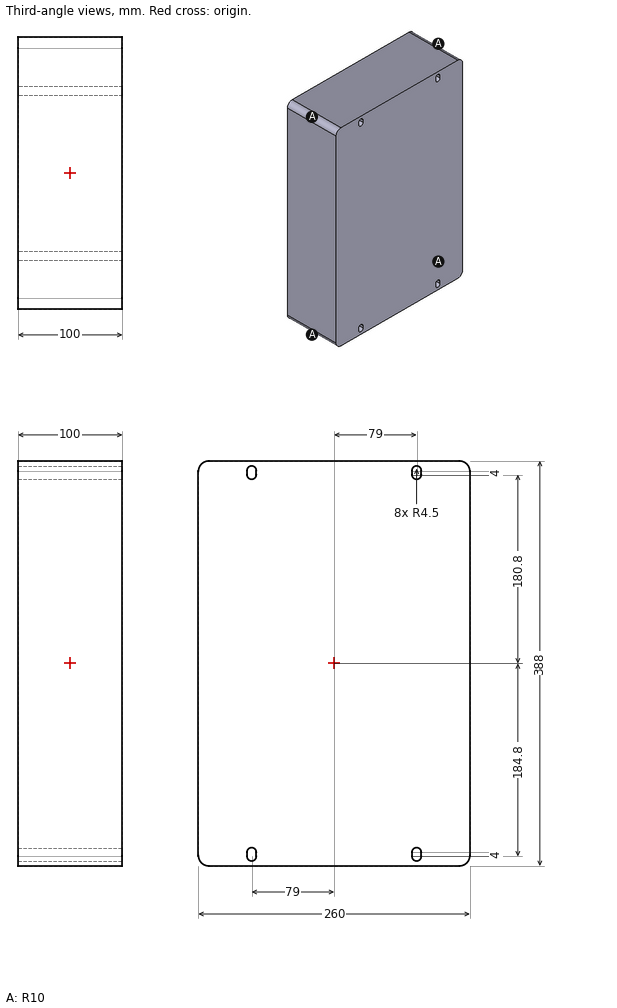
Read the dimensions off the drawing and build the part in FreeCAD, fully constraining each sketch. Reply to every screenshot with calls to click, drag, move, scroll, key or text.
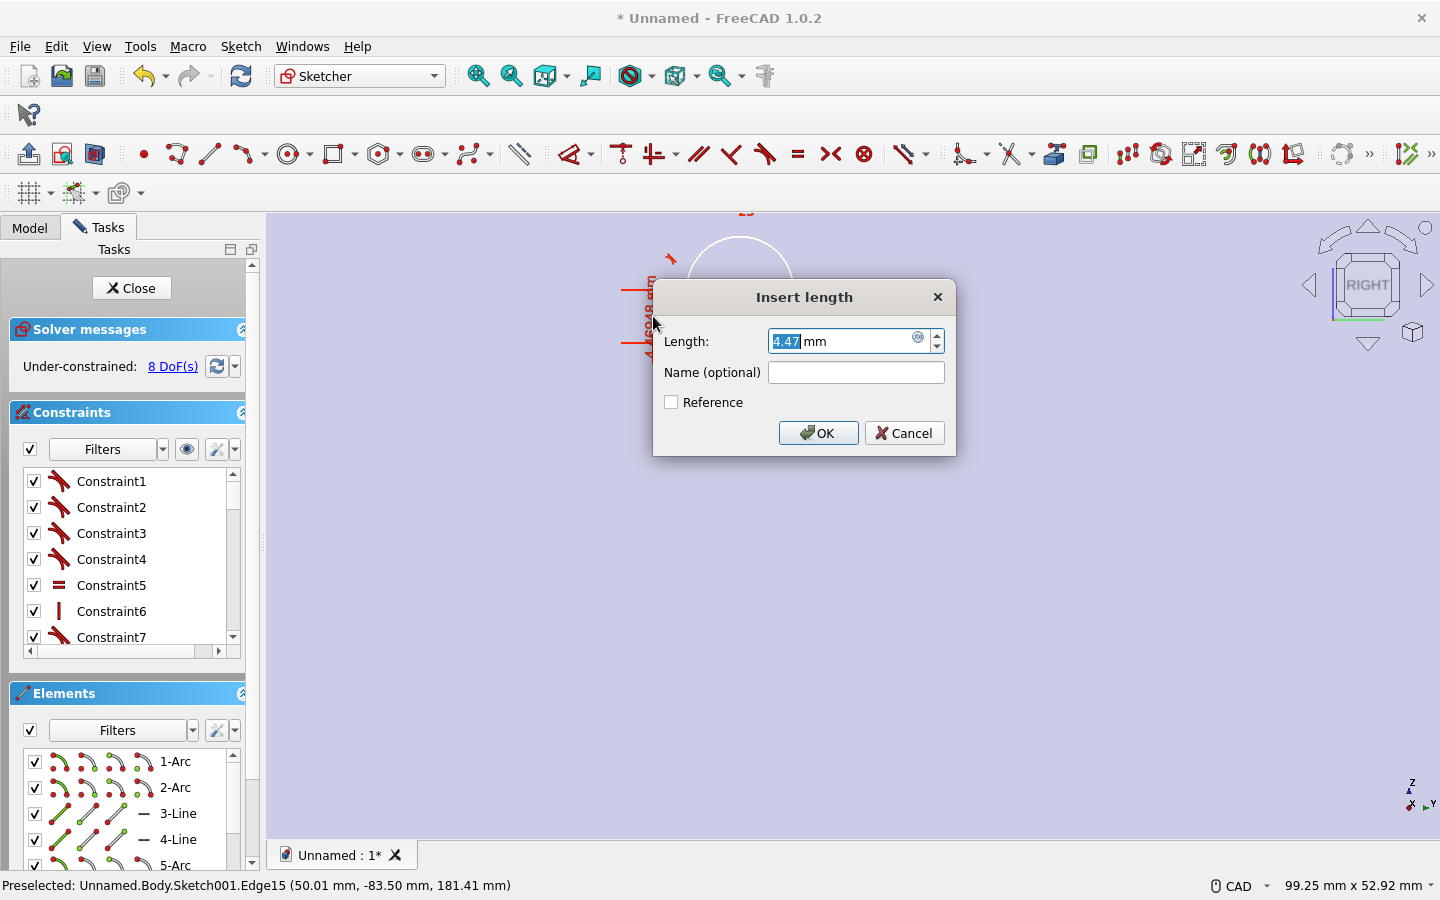
text(4)
key(Return)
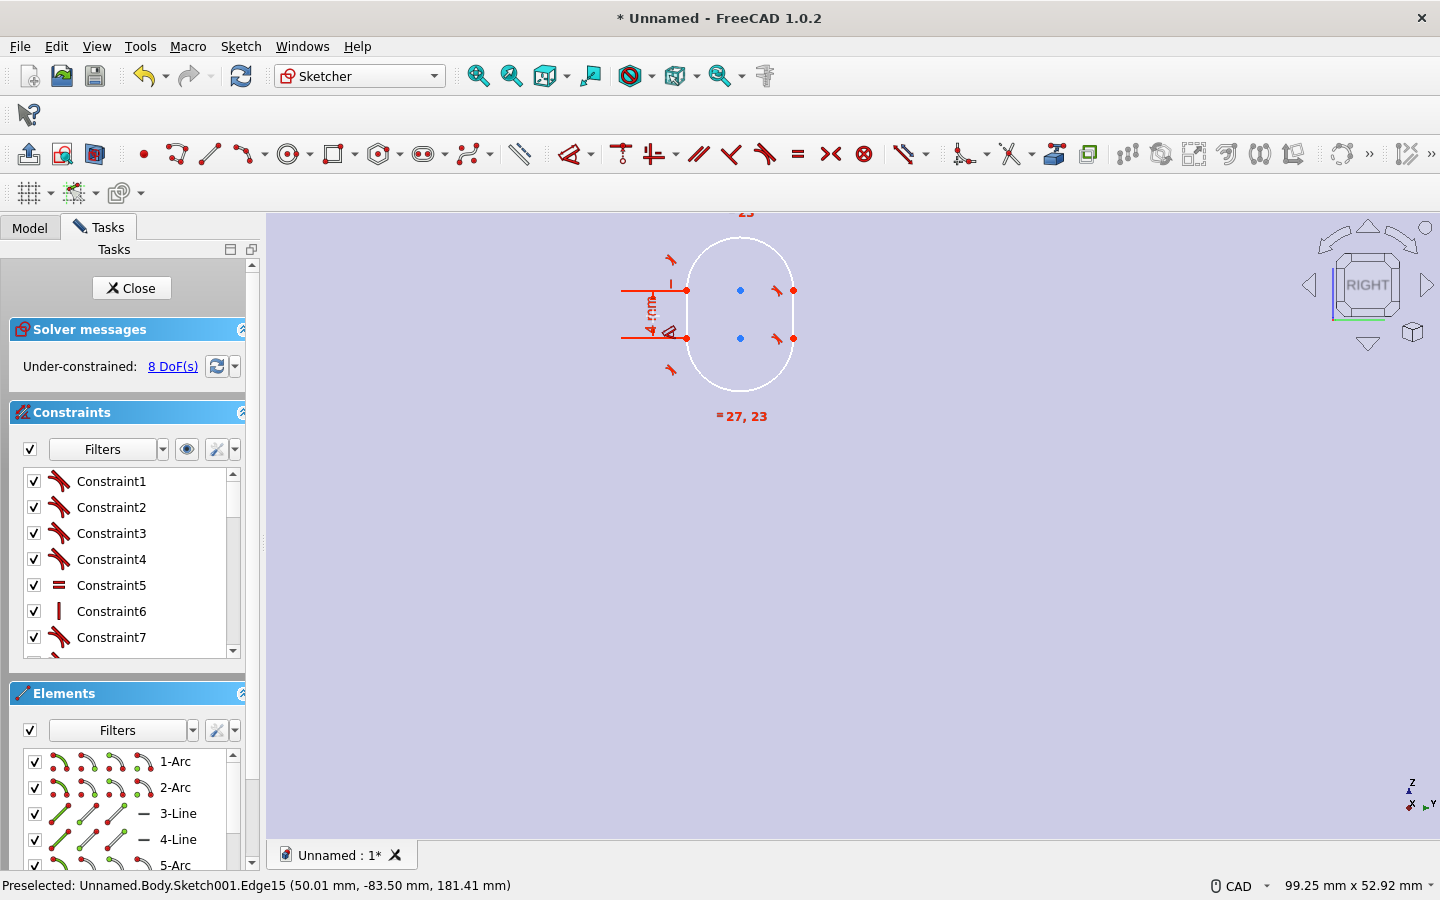
scroll(696, 332, down, 12)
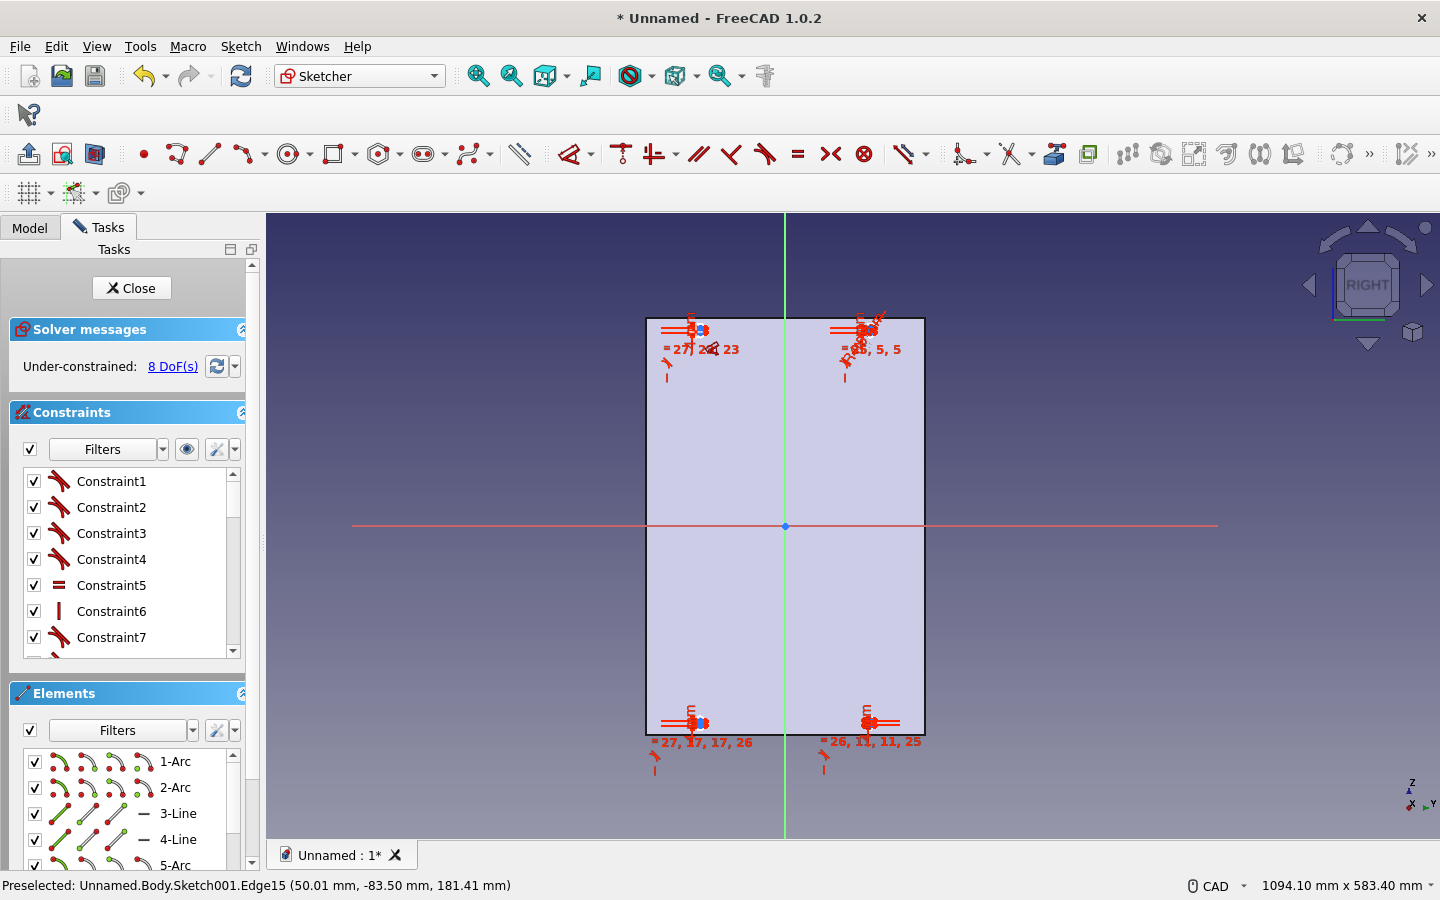
scroll(870, 333, up, 6)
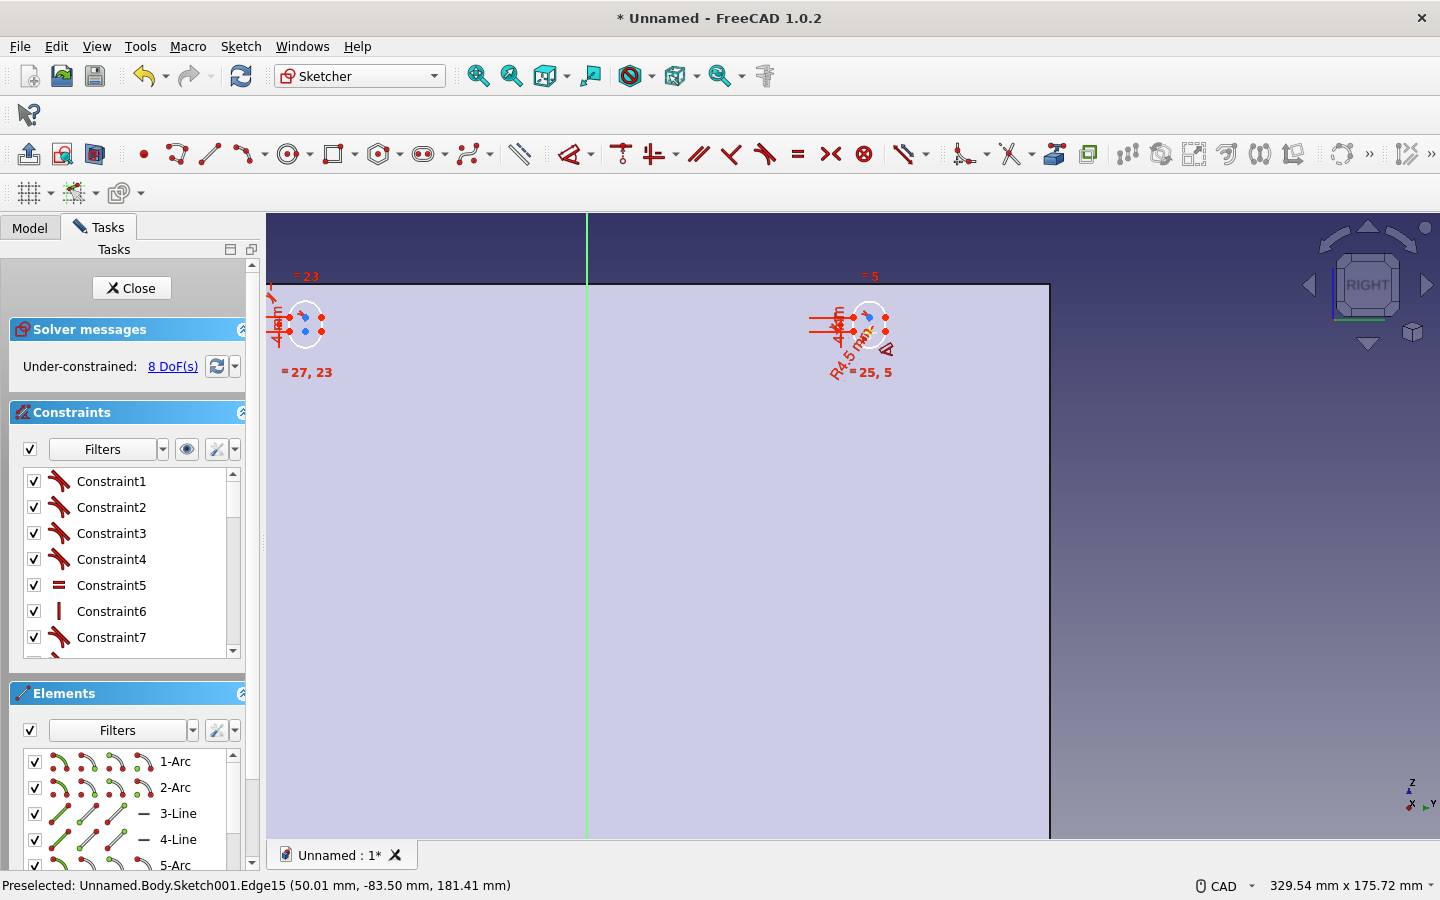
click(869, 332)
click(728, 298)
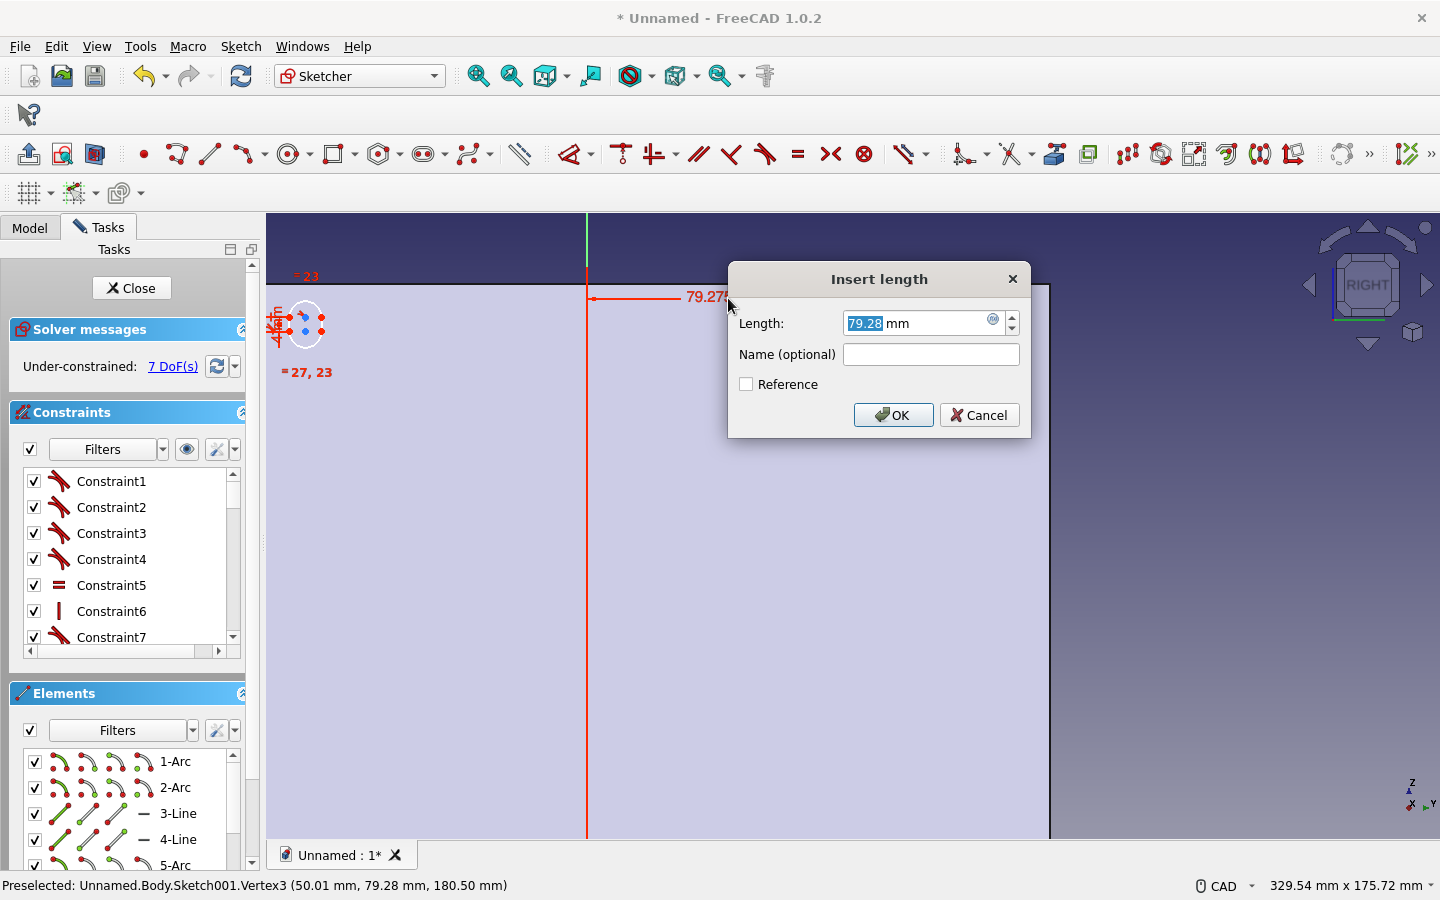
text(79)
key(Return)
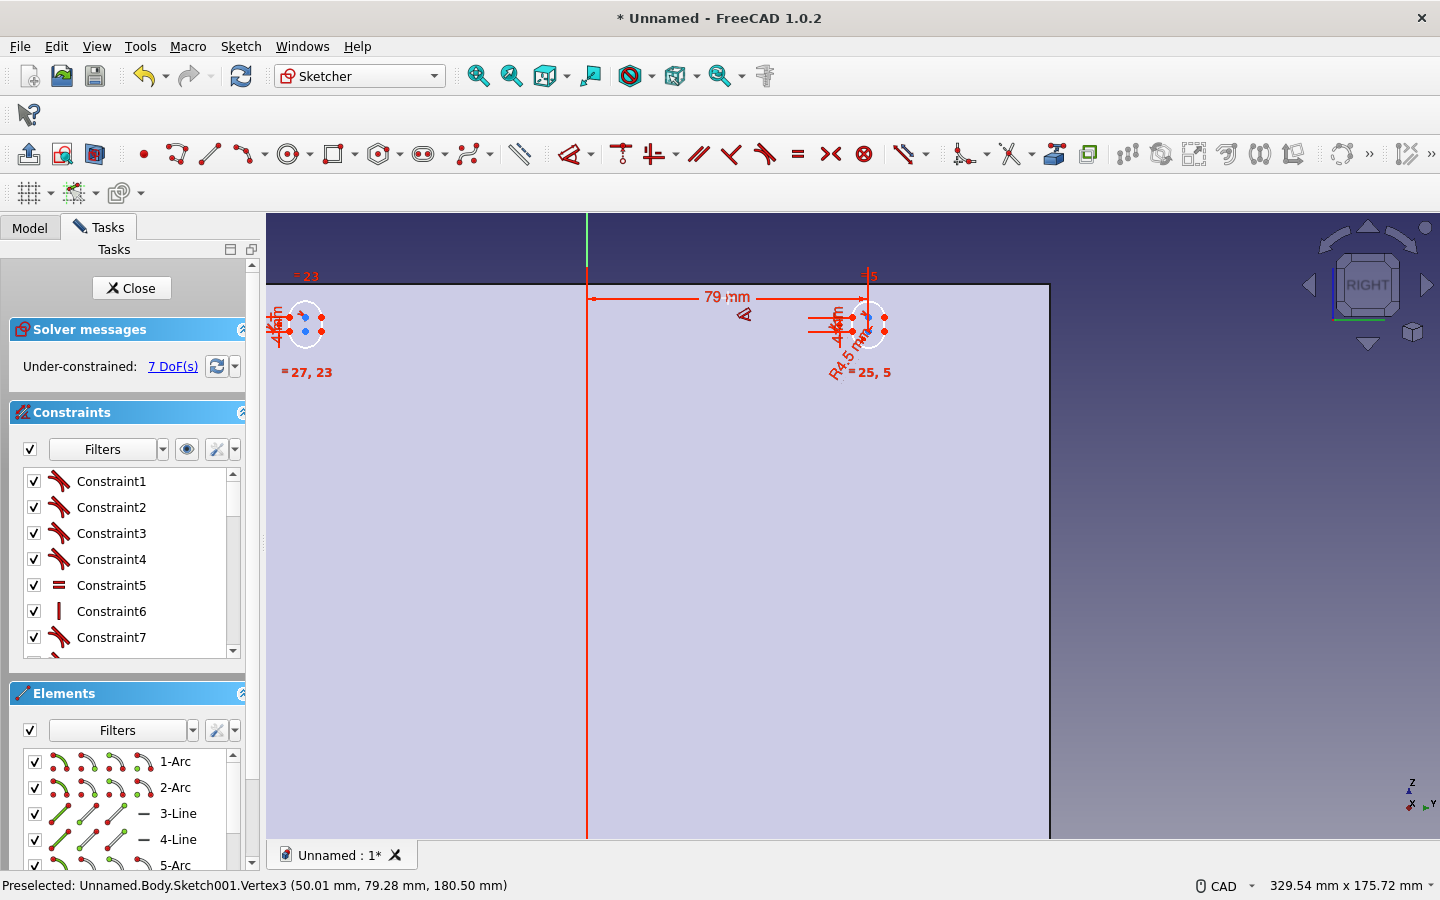
scroll(870, 333, down, 6)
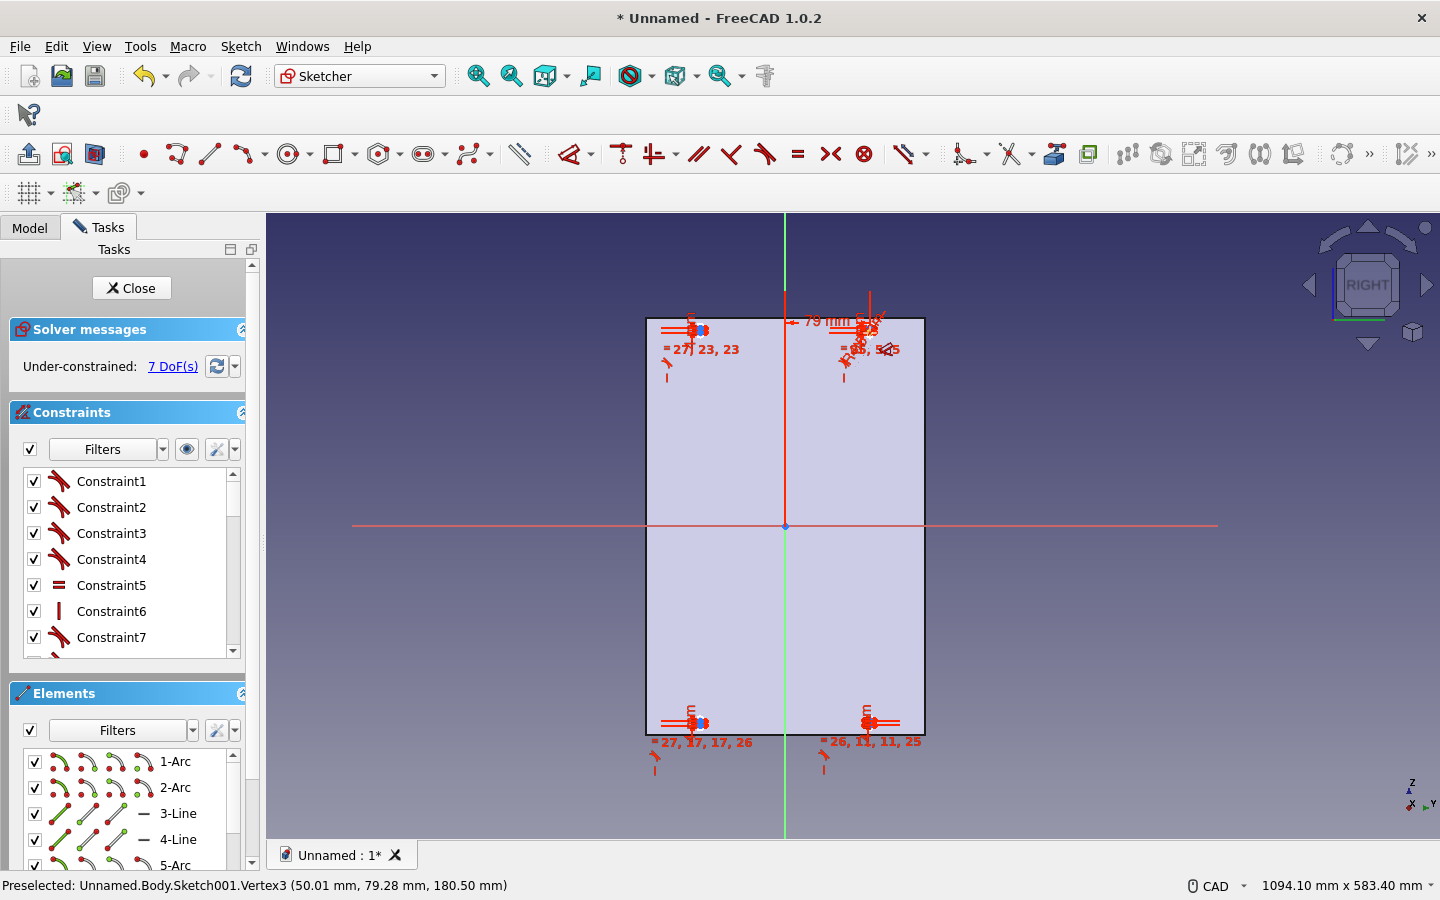
scroll(870, 725, up, 6)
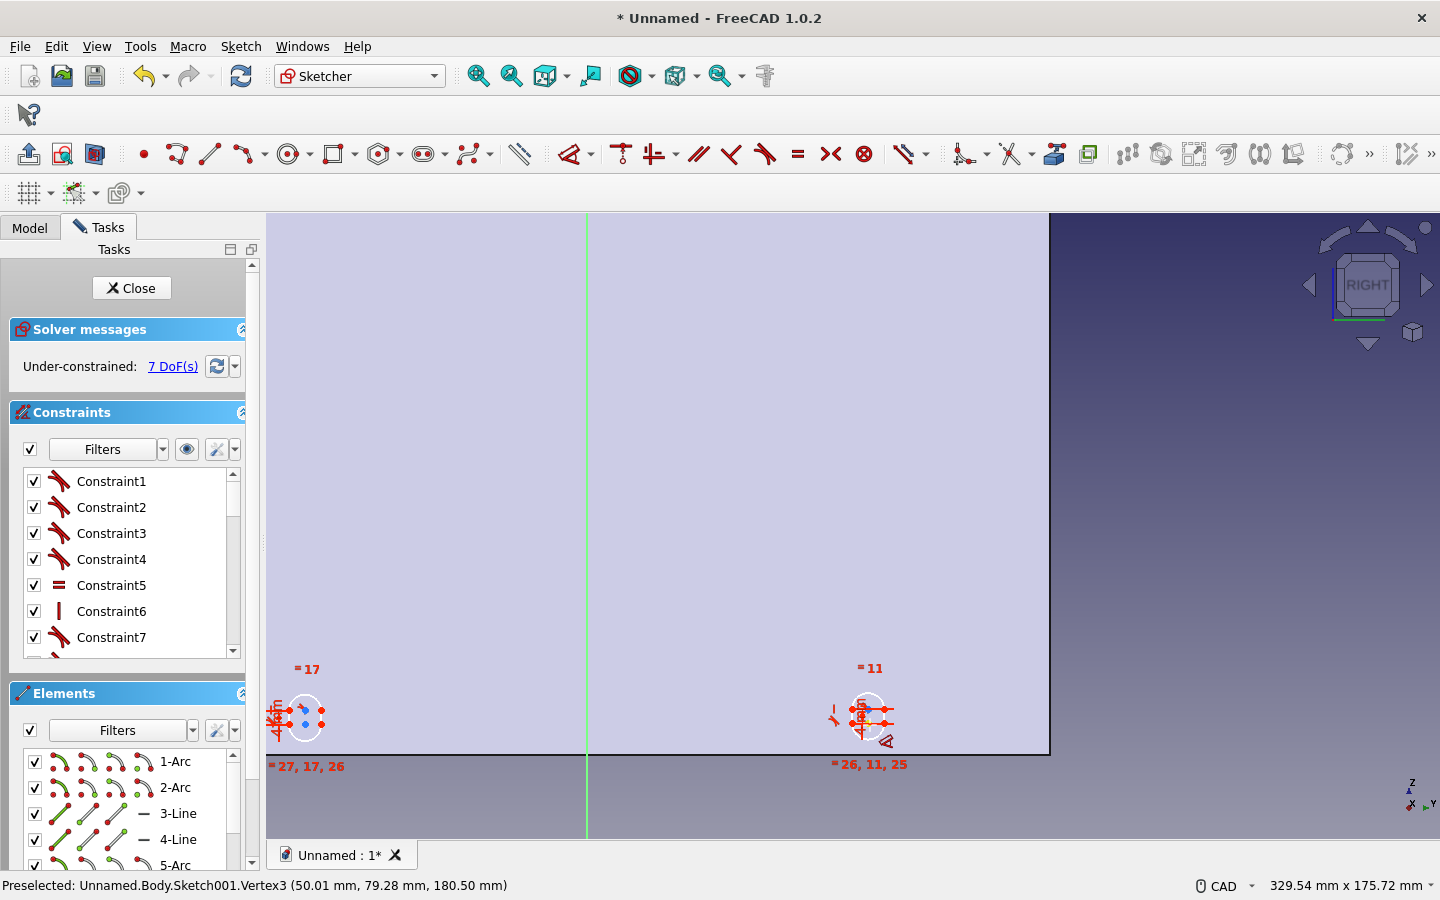
click(868, 724)
click(728, 758)